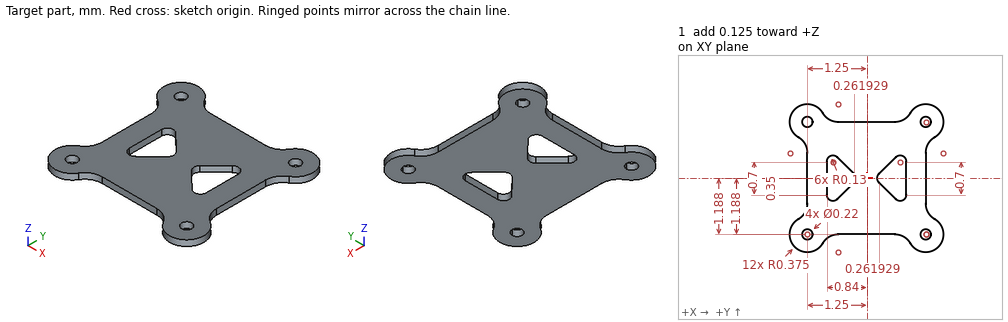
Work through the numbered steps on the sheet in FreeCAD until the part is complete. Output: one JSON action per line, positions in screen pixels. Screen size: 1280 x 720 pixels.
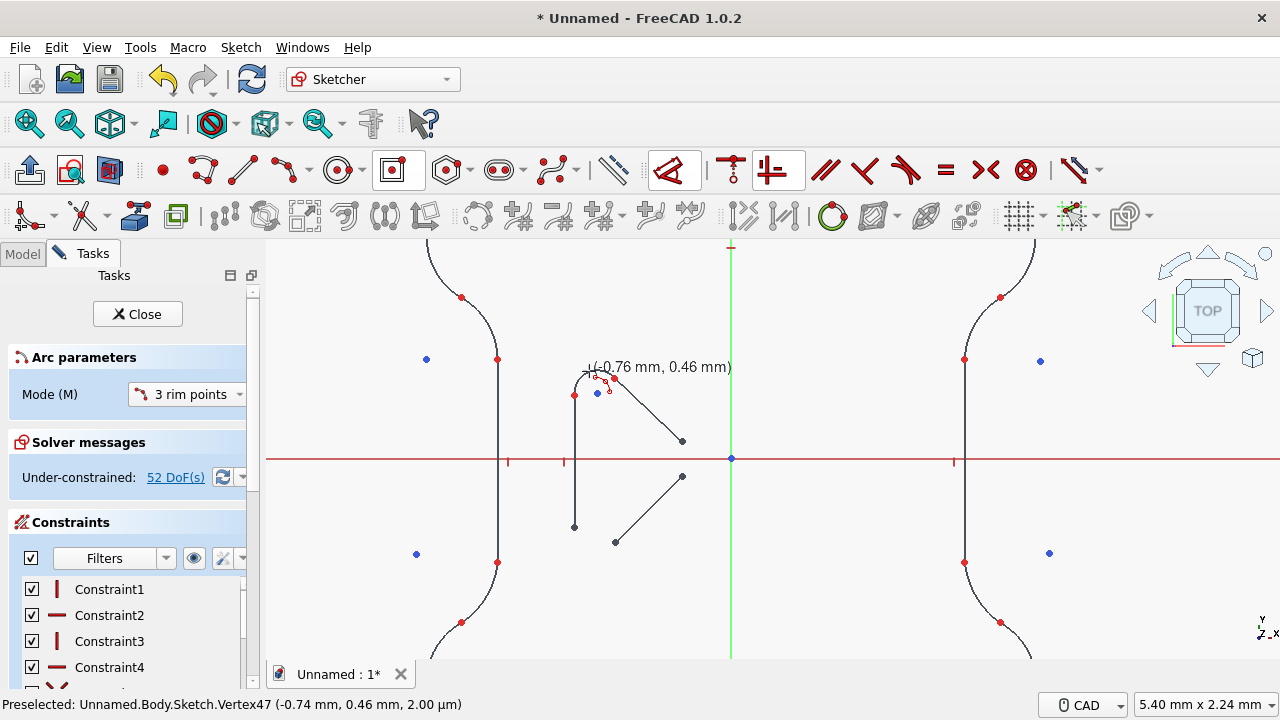
{"action": "left_click", "coordinate": [682, 442]}
{"action": "left_click", "coordinate": [682, 477]}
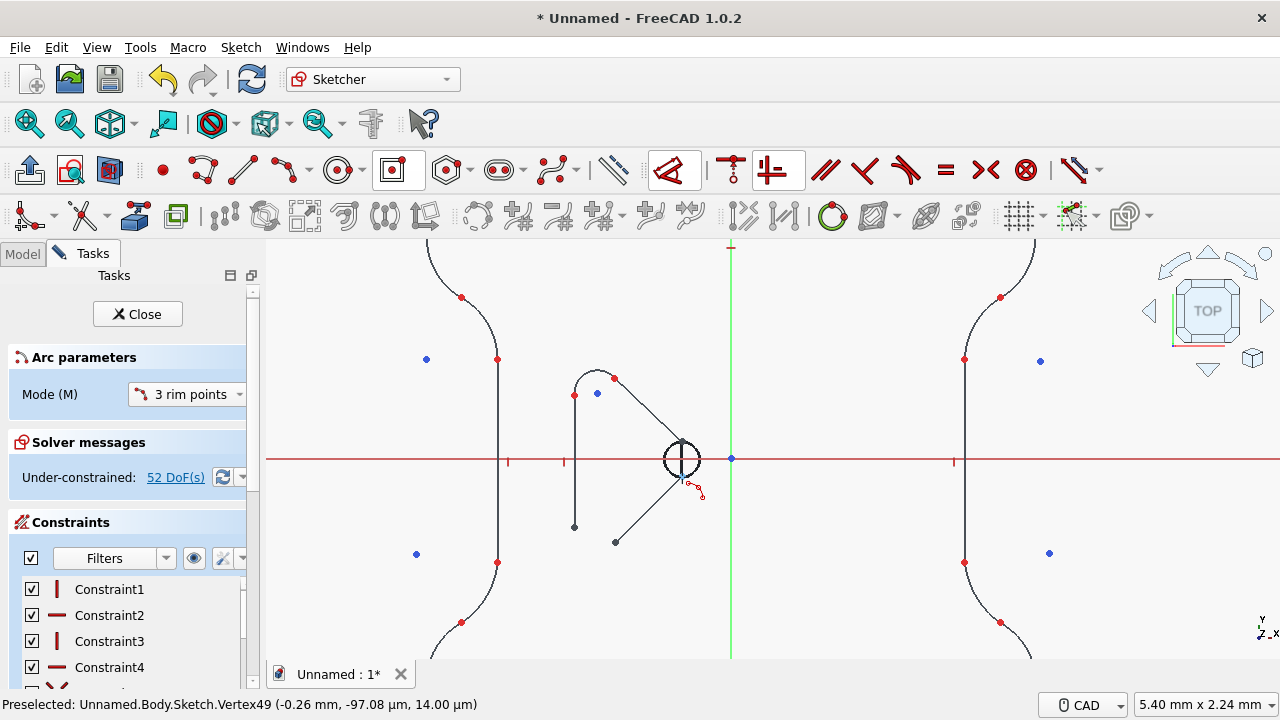
{"action": "scroll", "coordinate": [688, 466], "scroll_direction": "up", "scroll_amount": 5}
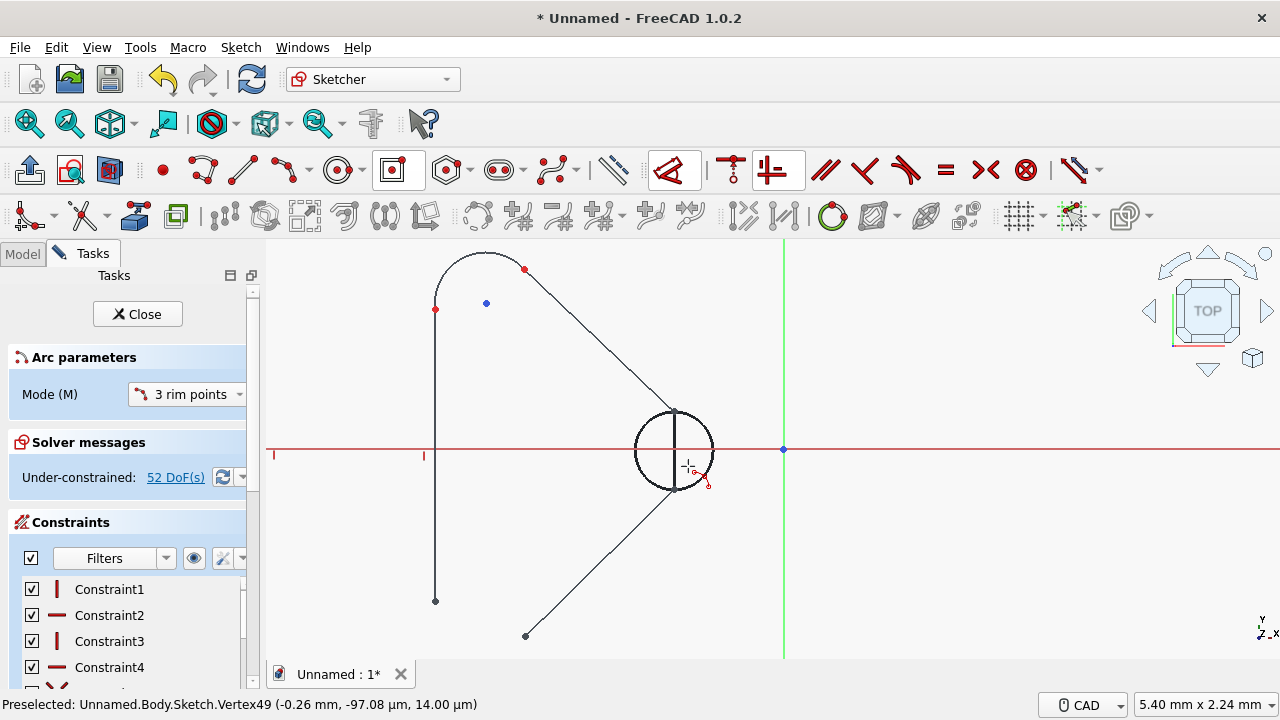
{"action": "left_click", "coordinate": [688, 466]}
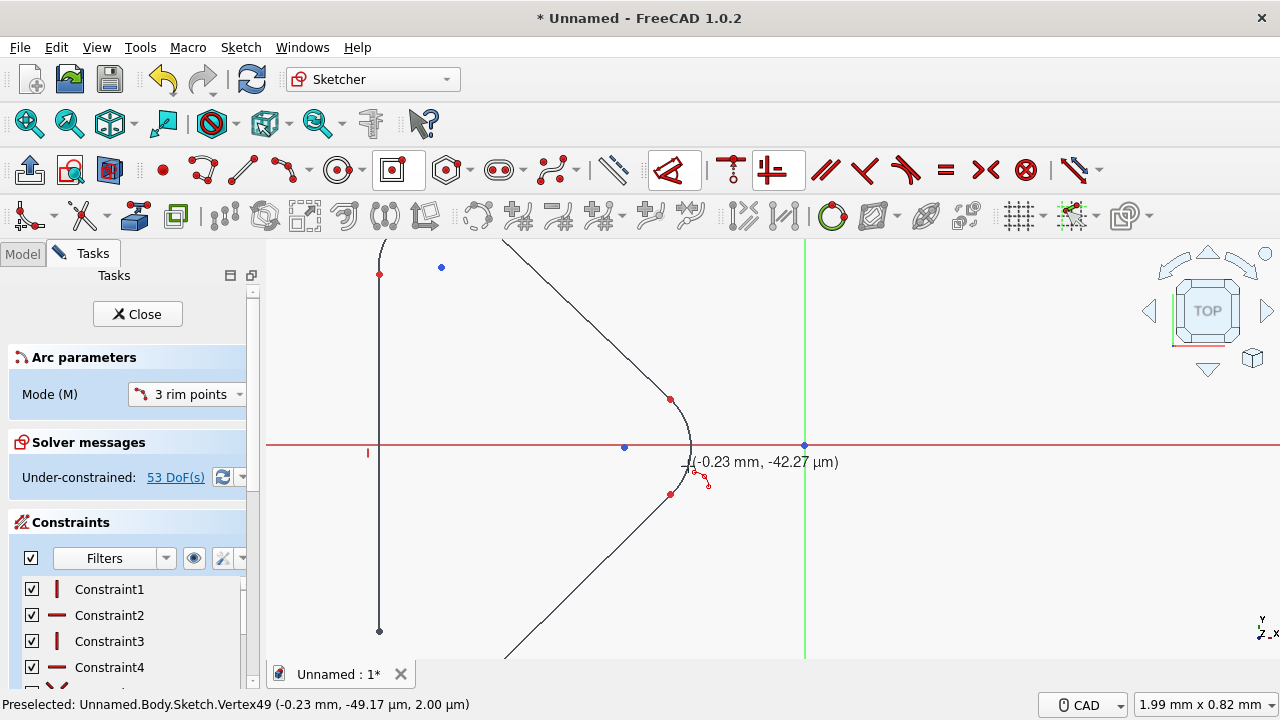
{"action": "scroll", "coordinate": [685, 450], "scroll_direction": "down", "scroll_amount": 9}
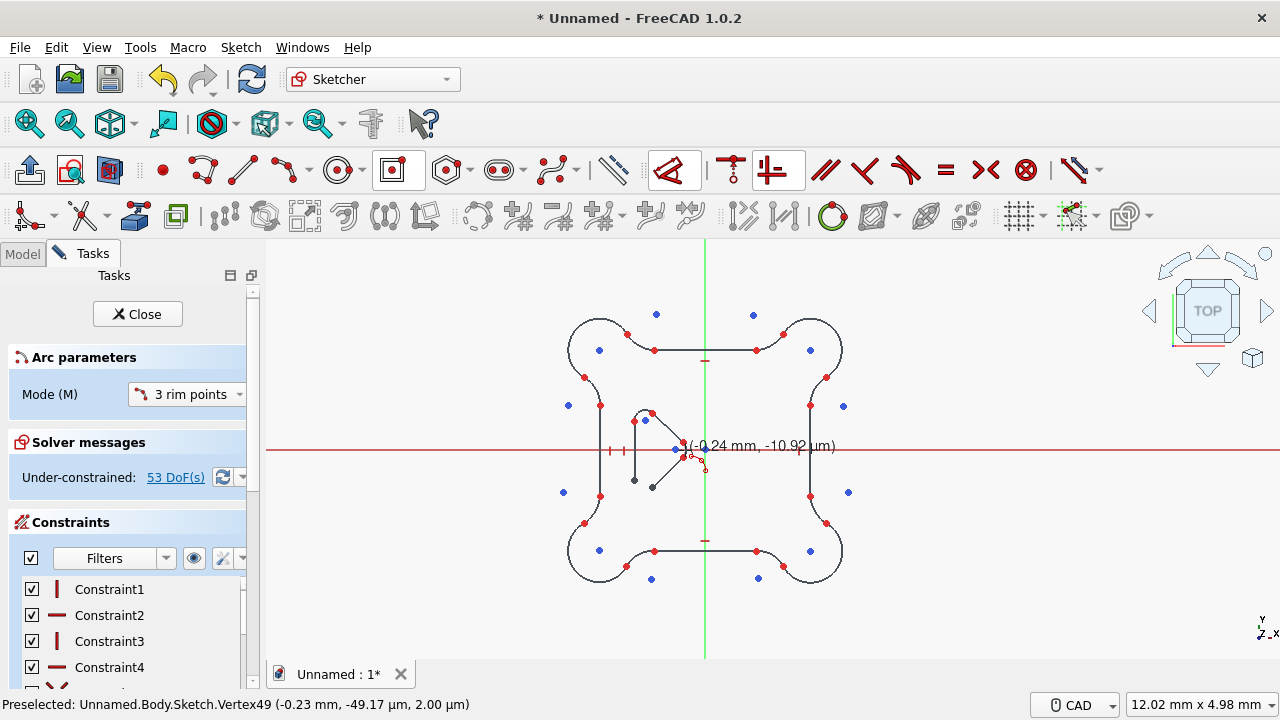
{"action": "left_click", "coordinate": [653, 488]}
{"action": "left_click", "coordinate": [635, 480]}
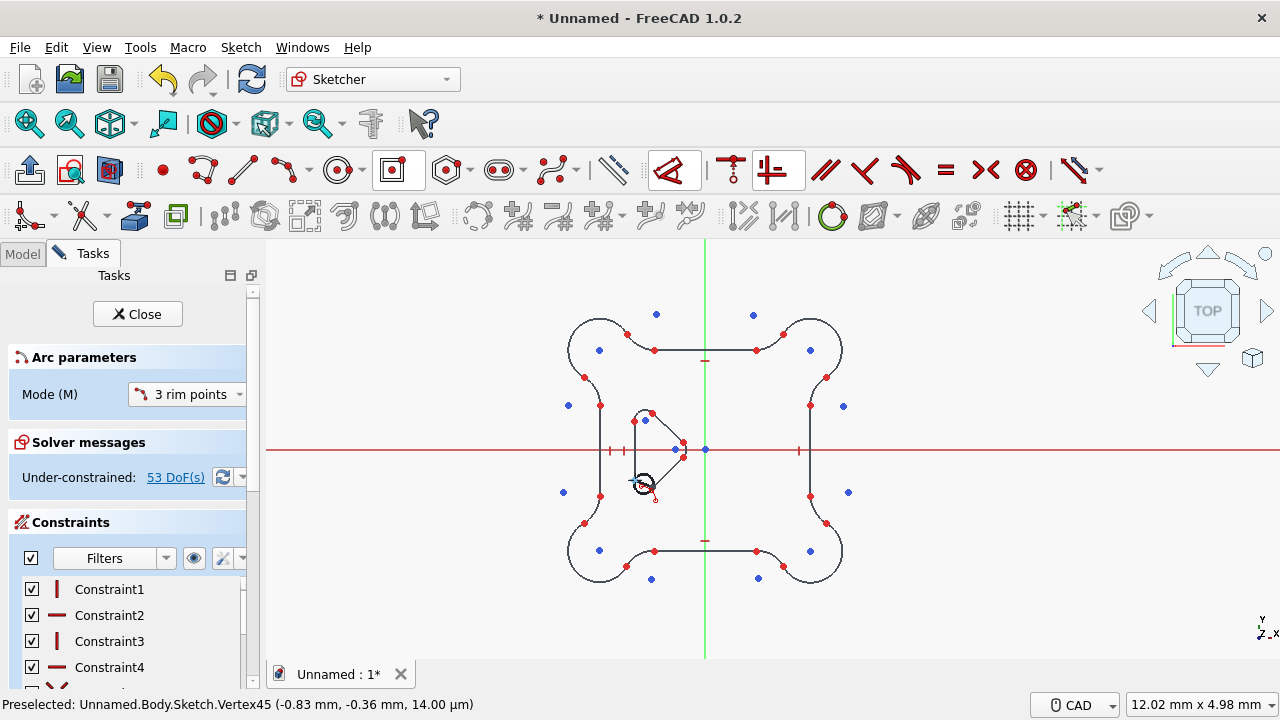
{"action": "scroll", "coordinate": [641, 489], "scroll_direction": "up", "scroll_amount": 5}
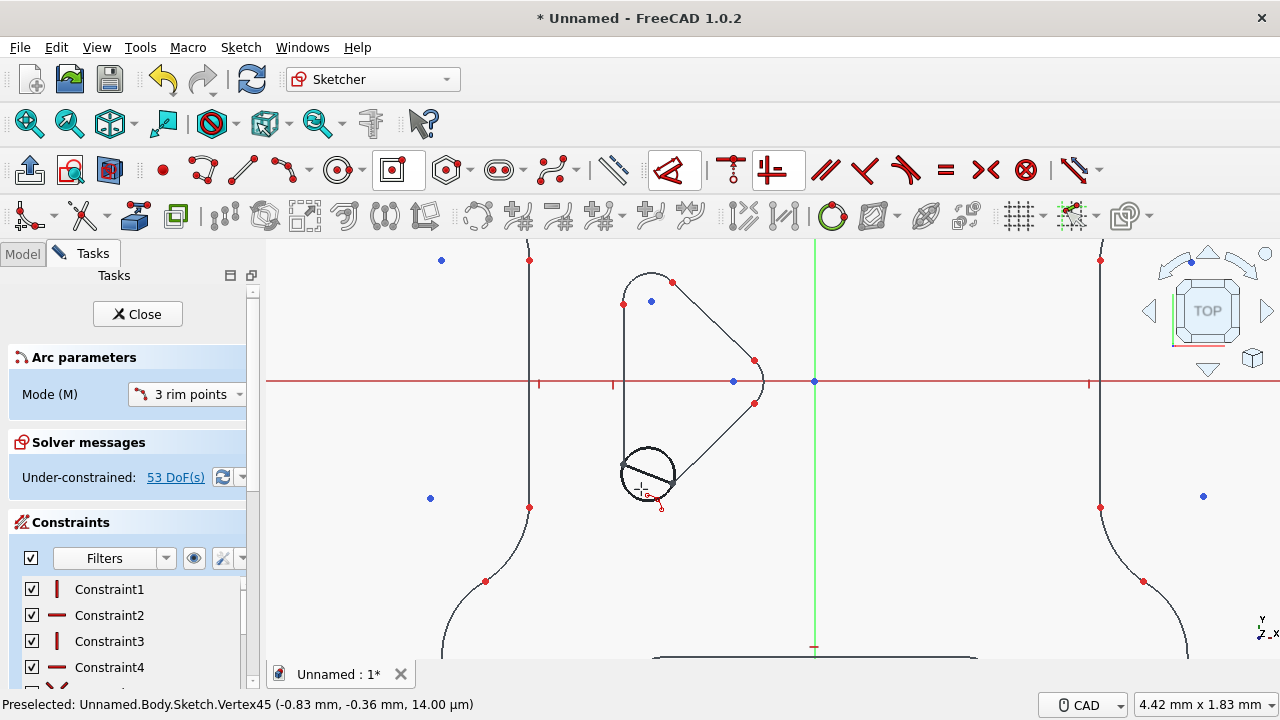
{"action": "left_click", "coordinate": [640, 489]}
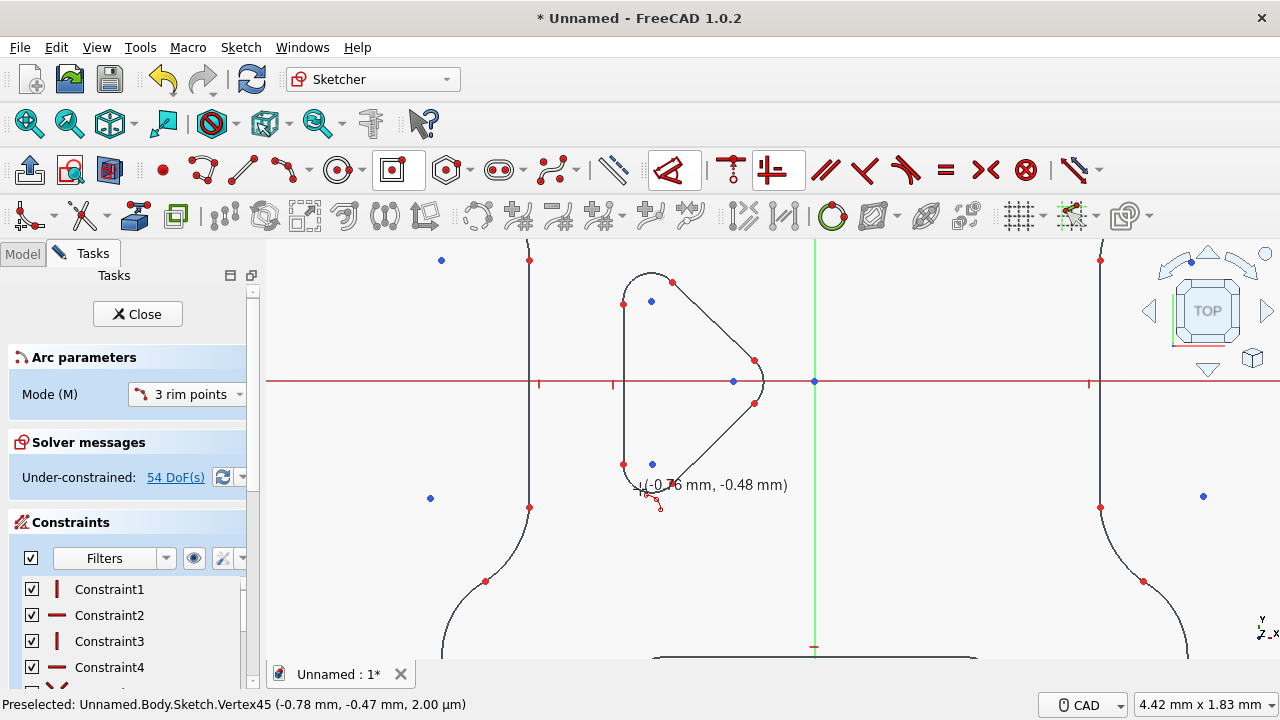
{"action": "left_click", "coordinate": [244, 170]}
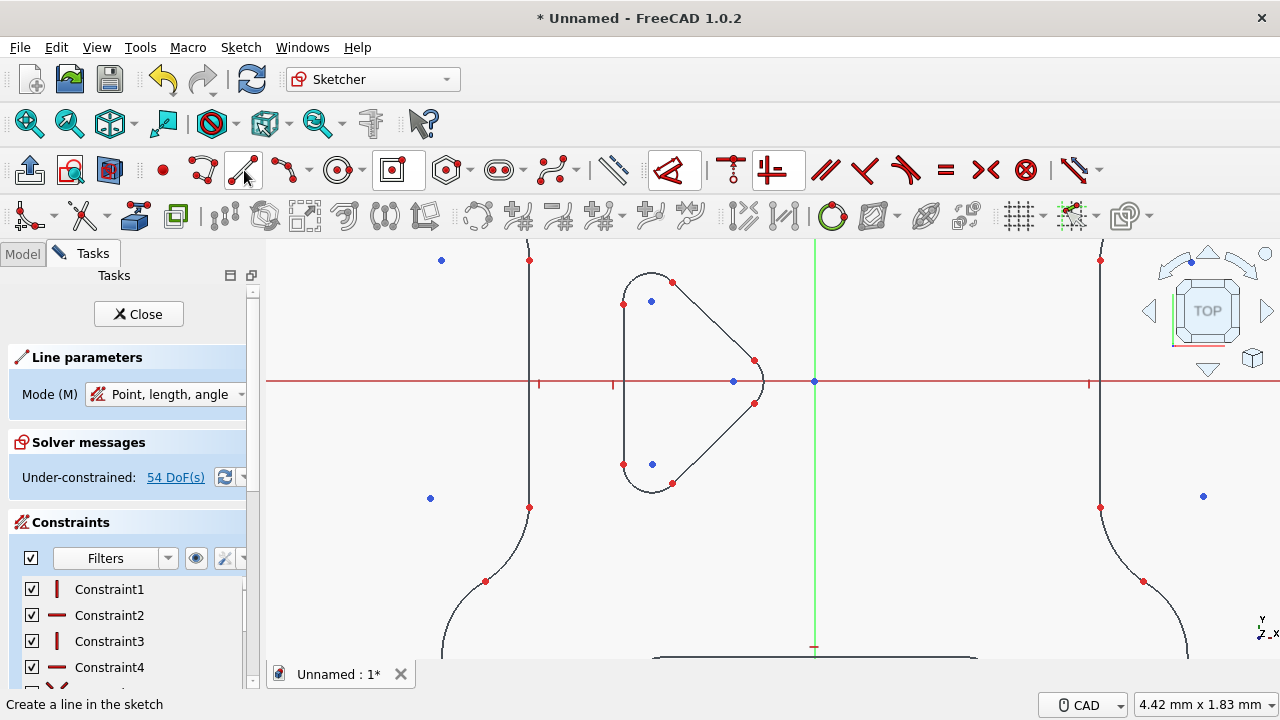
{"action": "left_click", "coordinate": [957, 483]}
{"action": "left_click", "coordinate": [875, 402]}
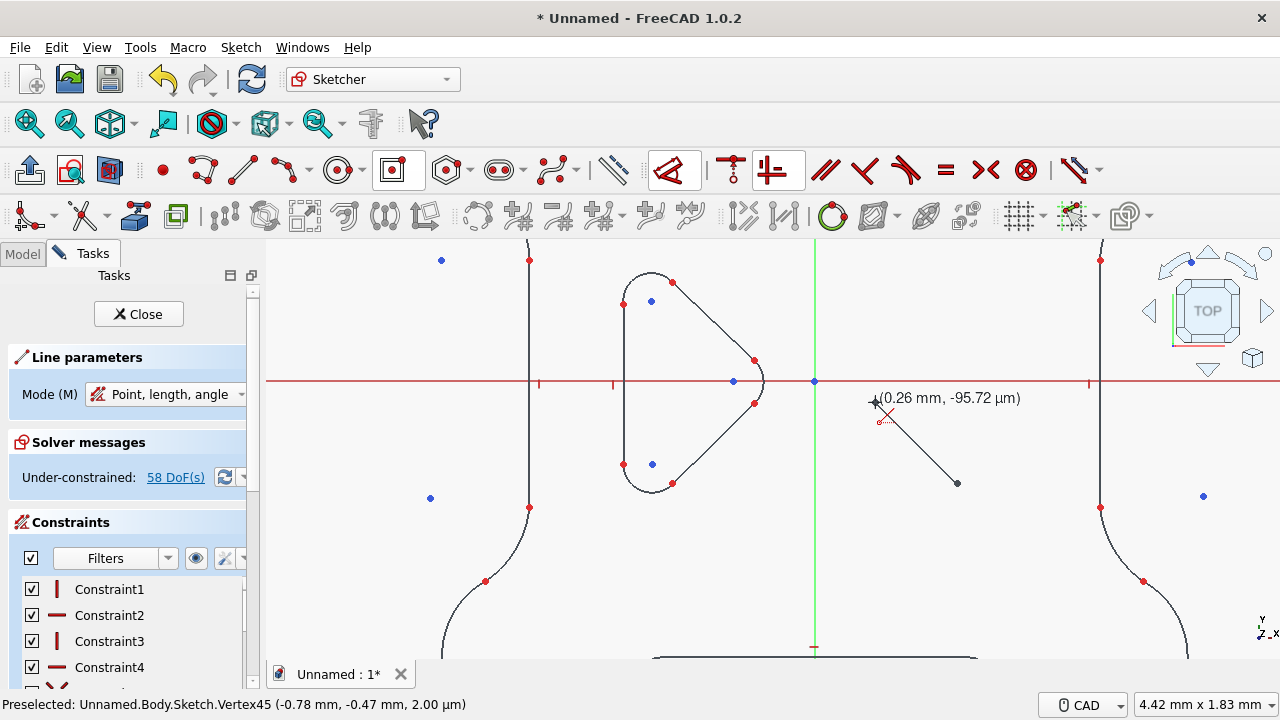
{"action": "left_click", "coordinate": [875, 360]}
{"action": "left_click", "coordinate": [957, 280]}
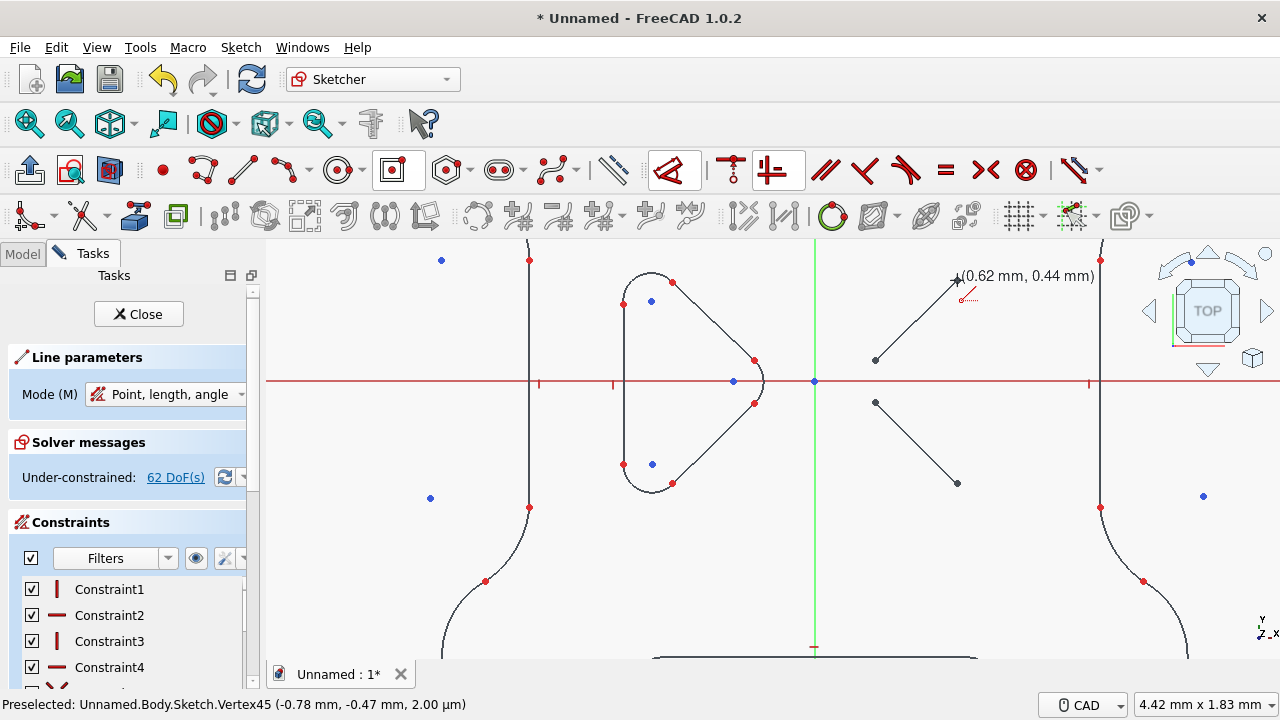
{"action": "left_click", "coordinate": [1007, 301]}
{"action": "left_click", "coordinate": [1007, 461]}